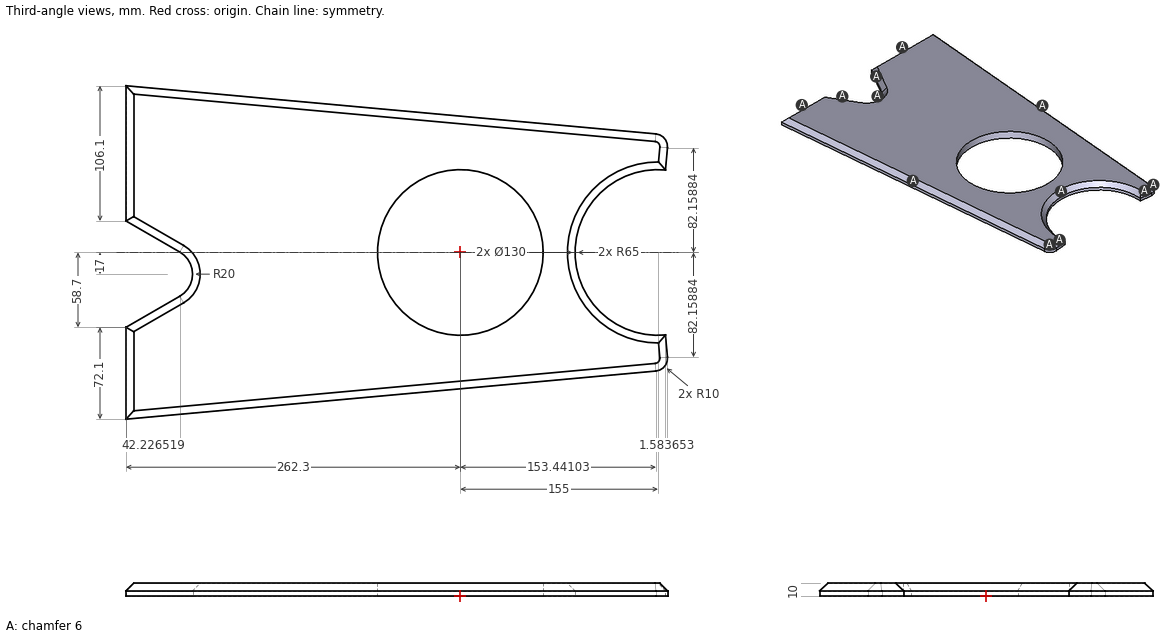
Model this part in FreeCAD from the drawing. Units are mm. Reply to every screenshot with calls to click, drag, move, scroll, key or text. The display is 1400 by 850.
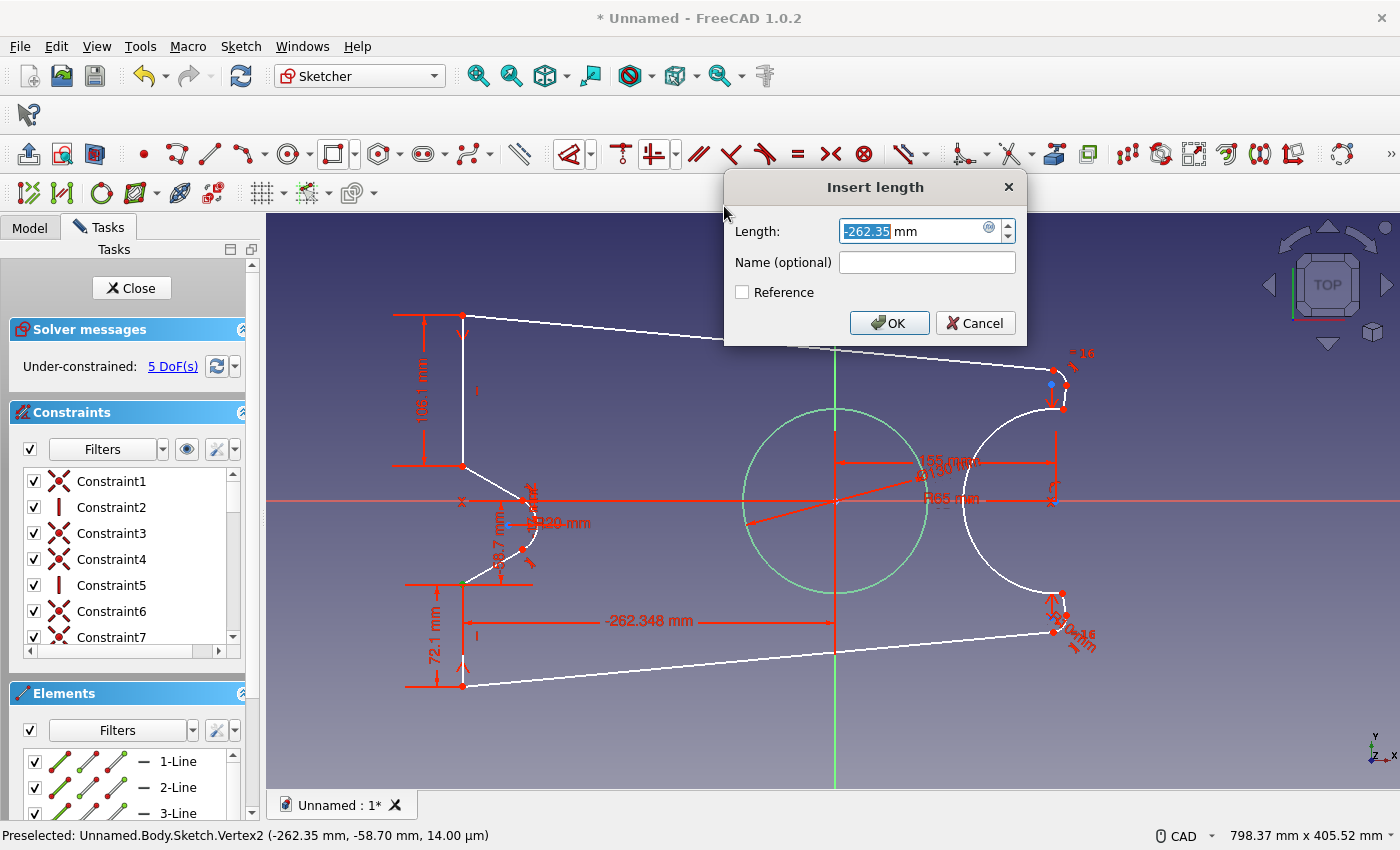
text(-262.3)
key(Return)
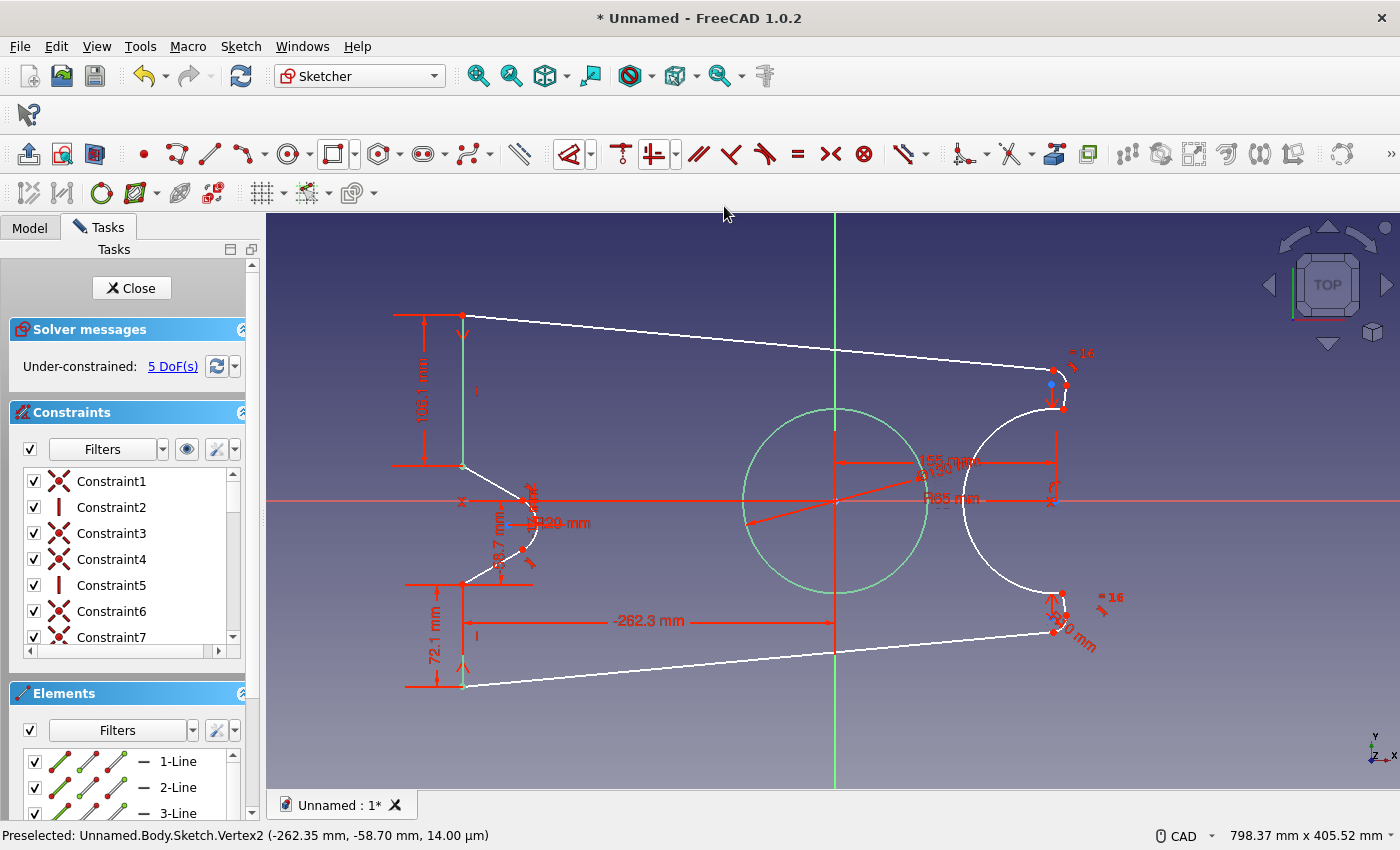
click(1066, 616)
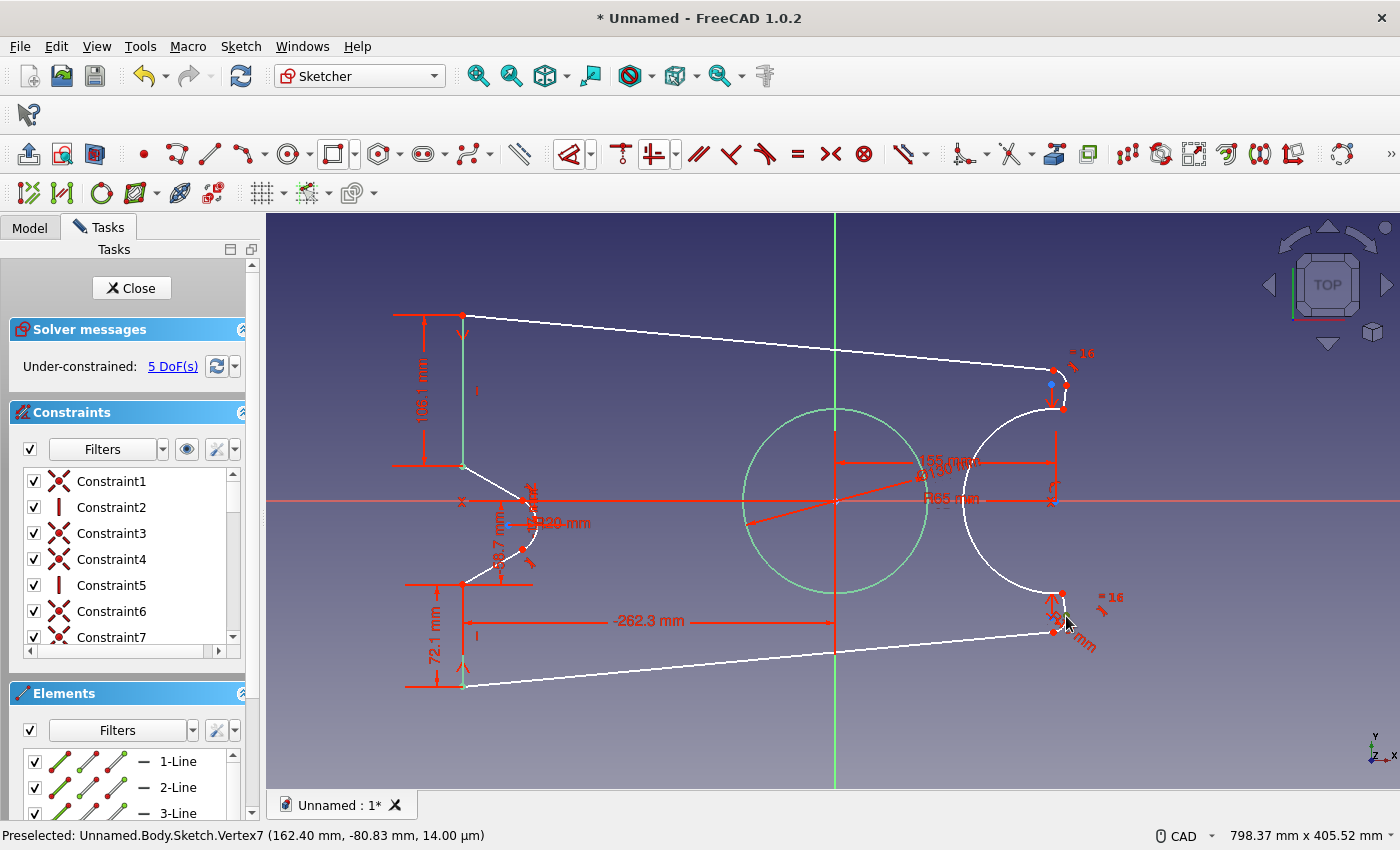
click(590, 154)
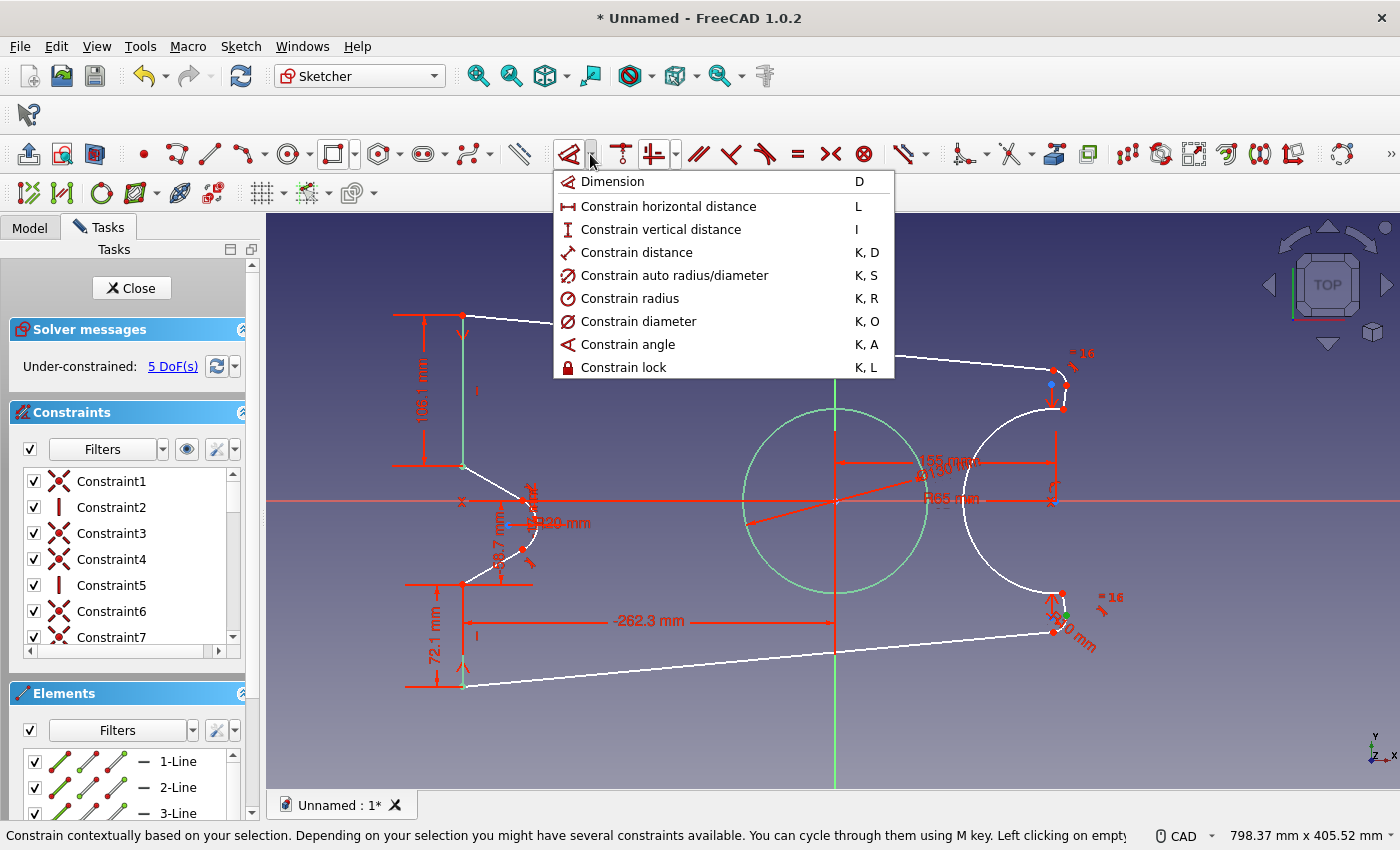
click(724, 230)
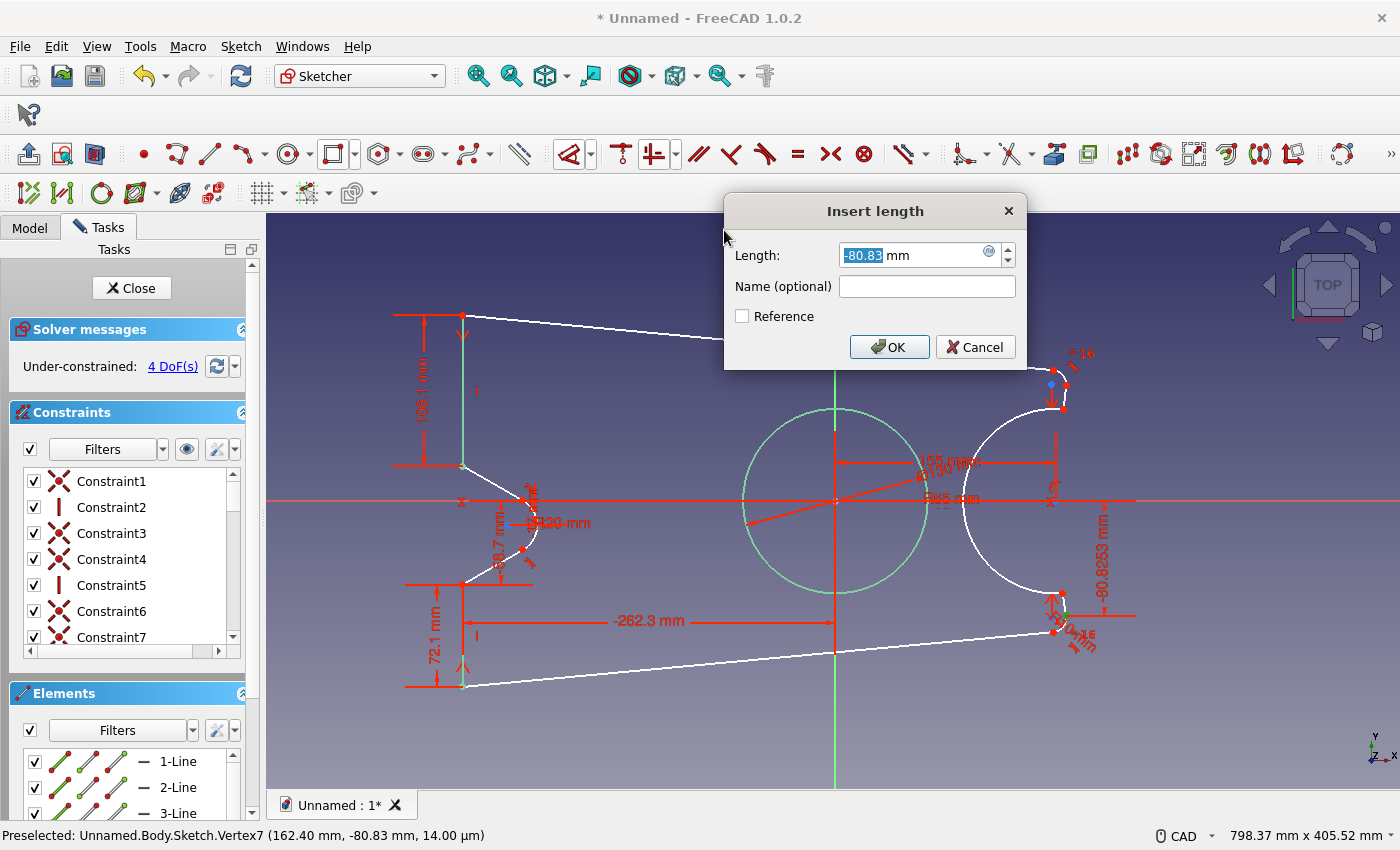
text(-82.15884)
key(Return)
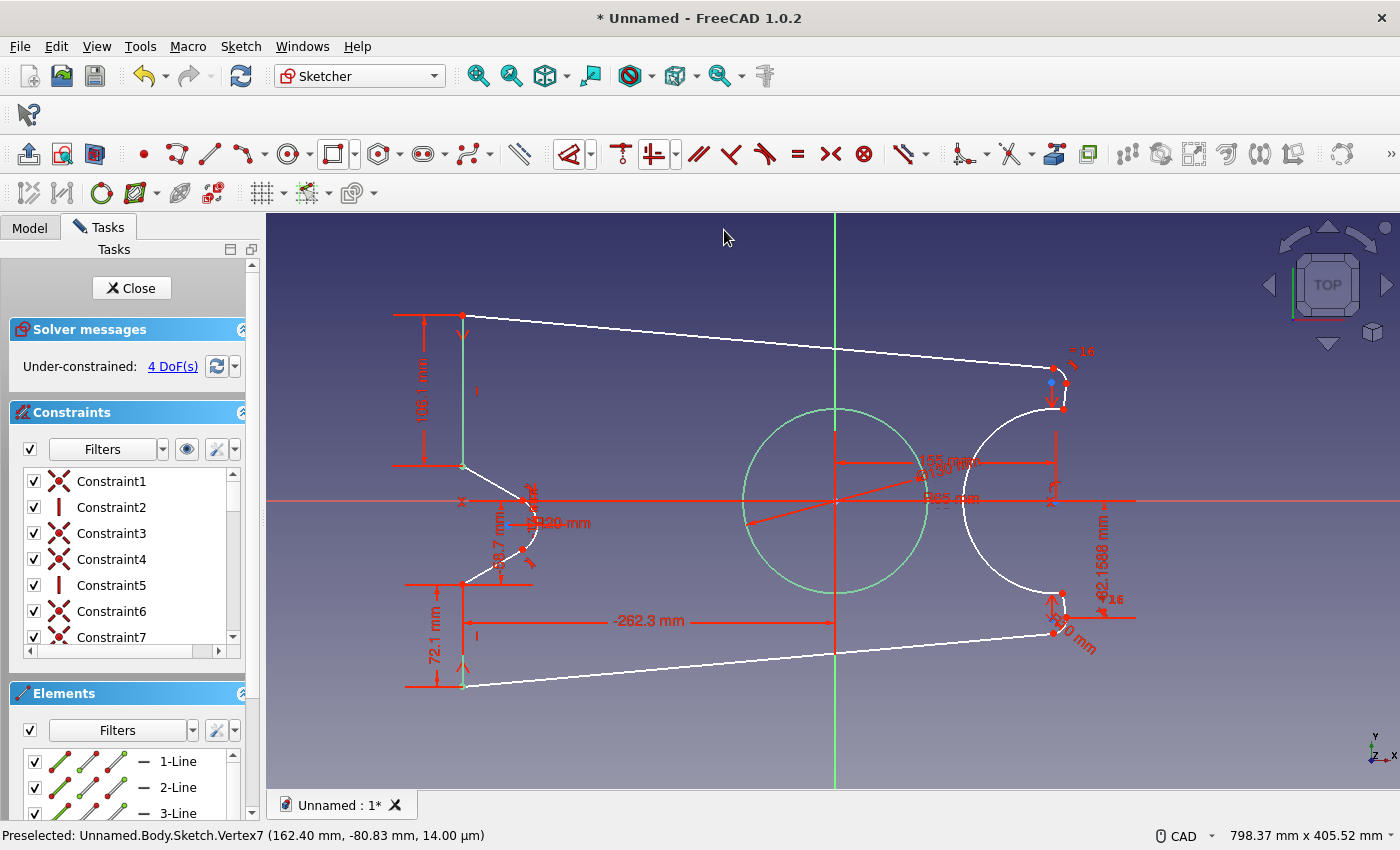
click(1066, 384)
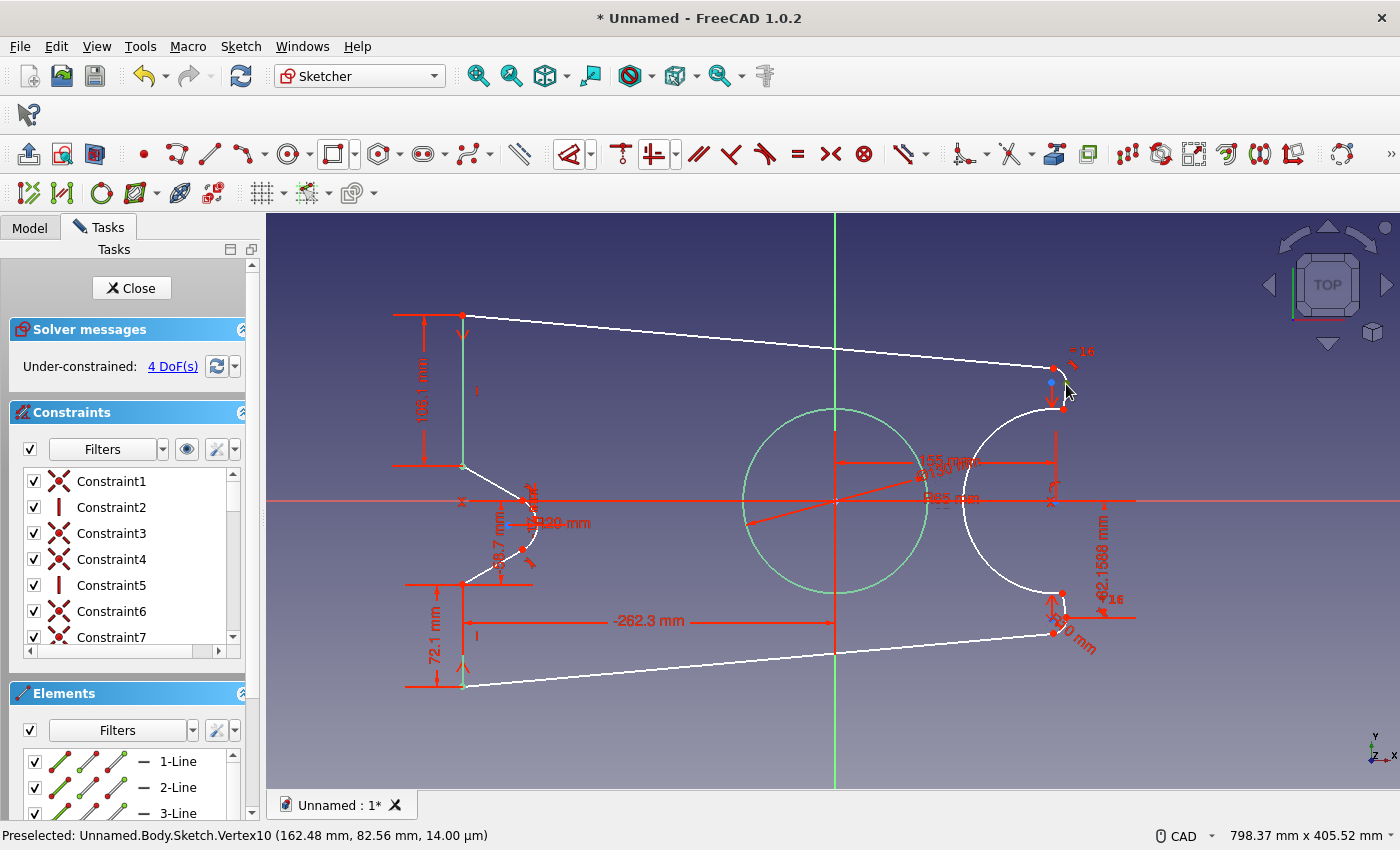
click(590, 154)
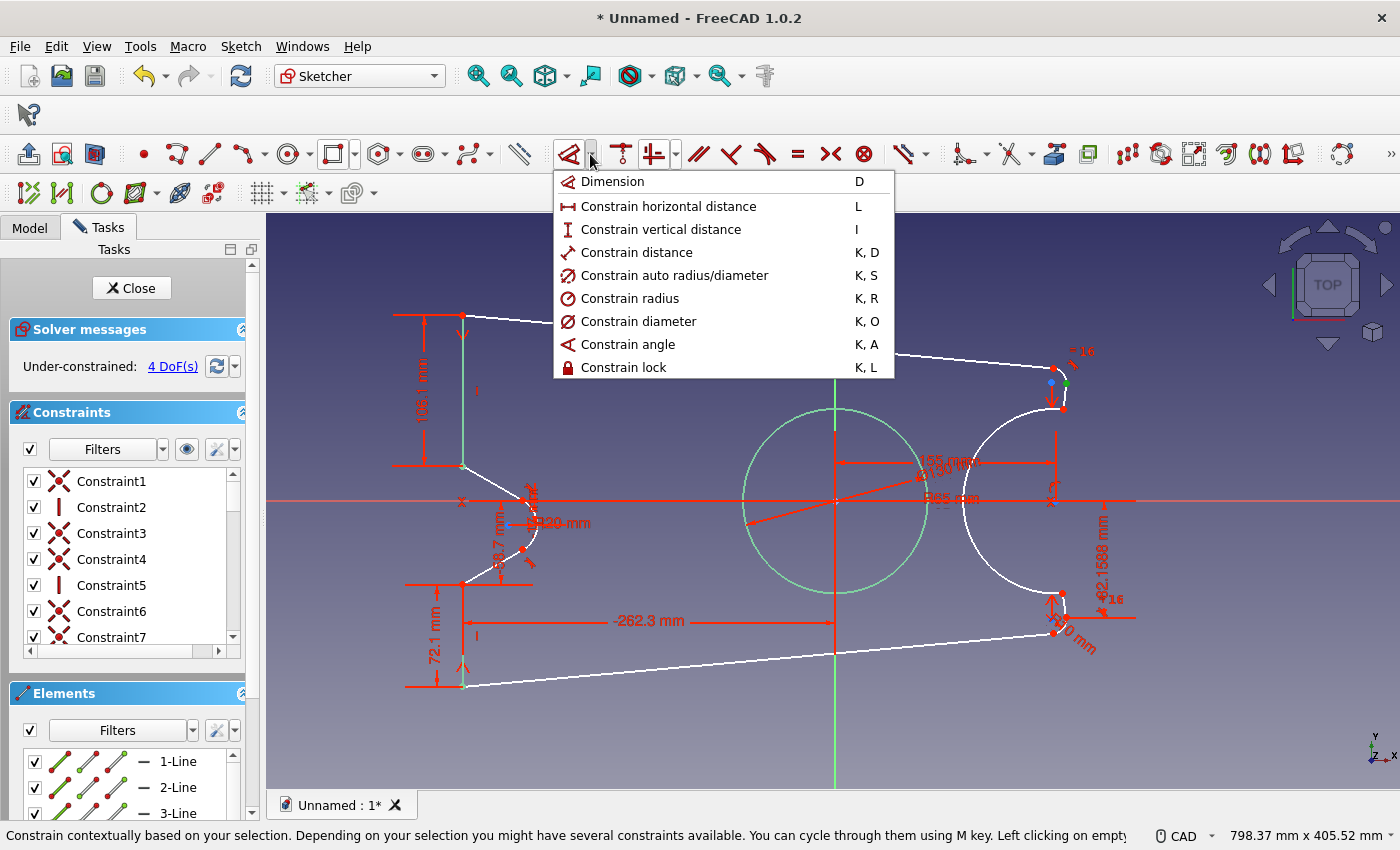
click(724, 230)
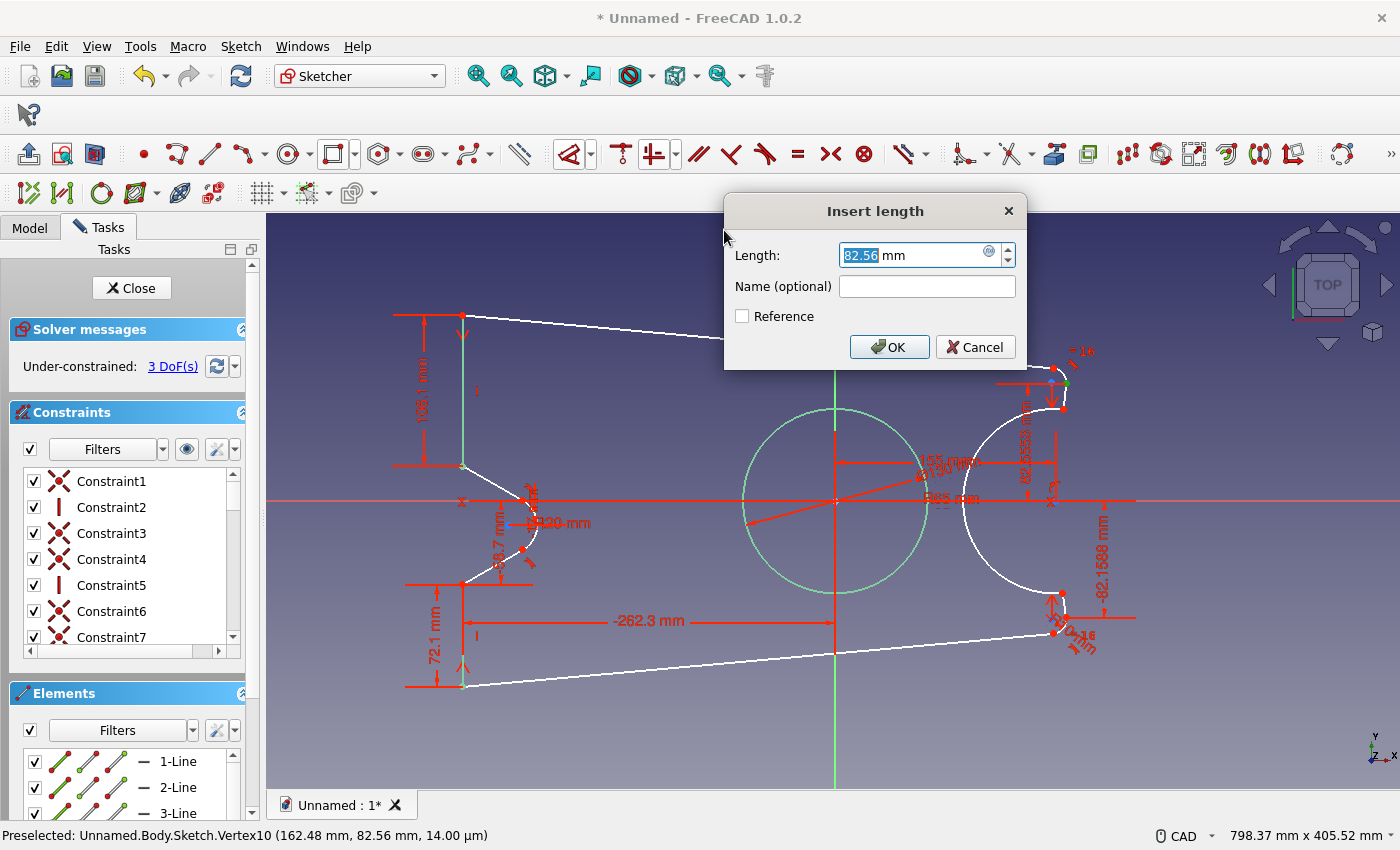
text(82.15884)
key(Return)